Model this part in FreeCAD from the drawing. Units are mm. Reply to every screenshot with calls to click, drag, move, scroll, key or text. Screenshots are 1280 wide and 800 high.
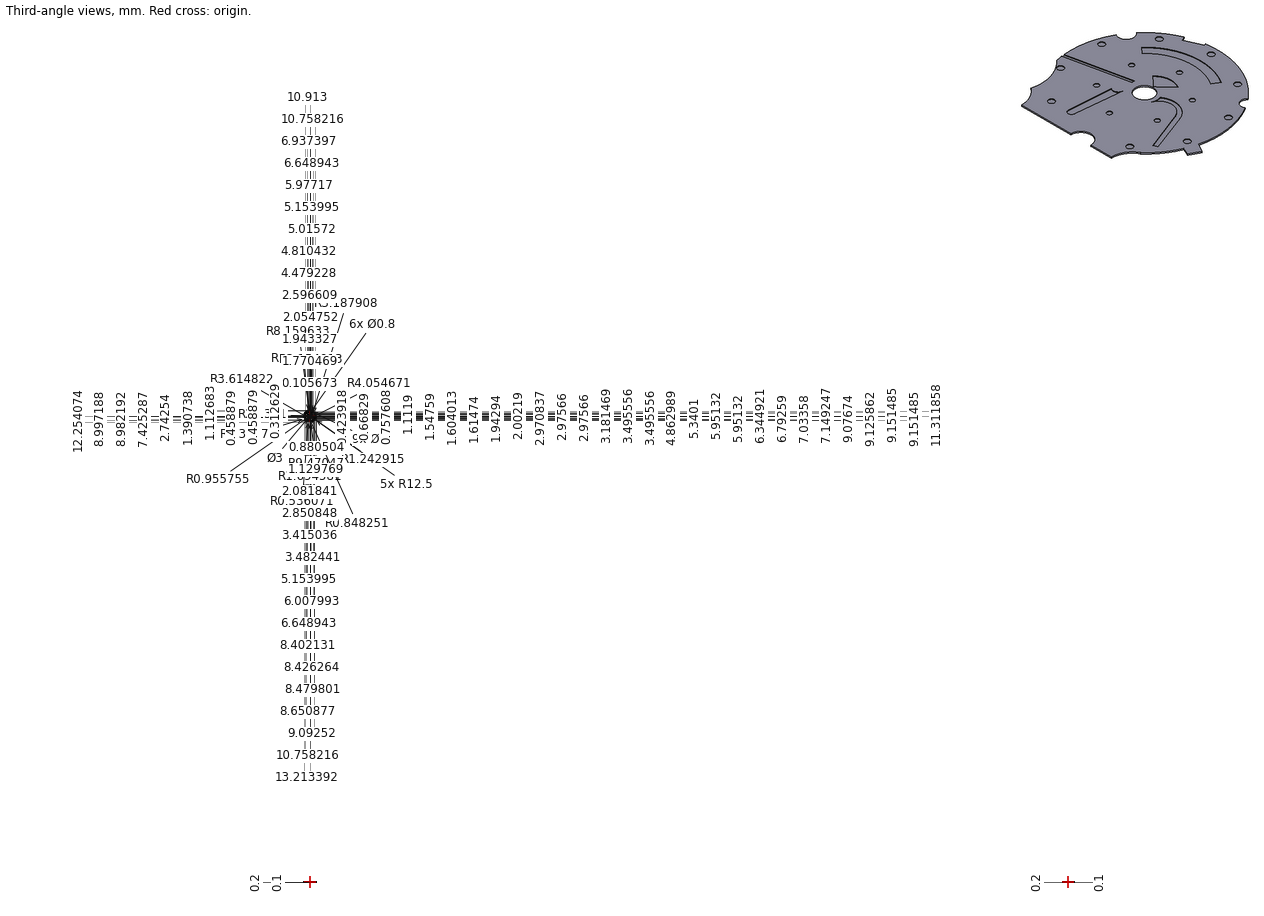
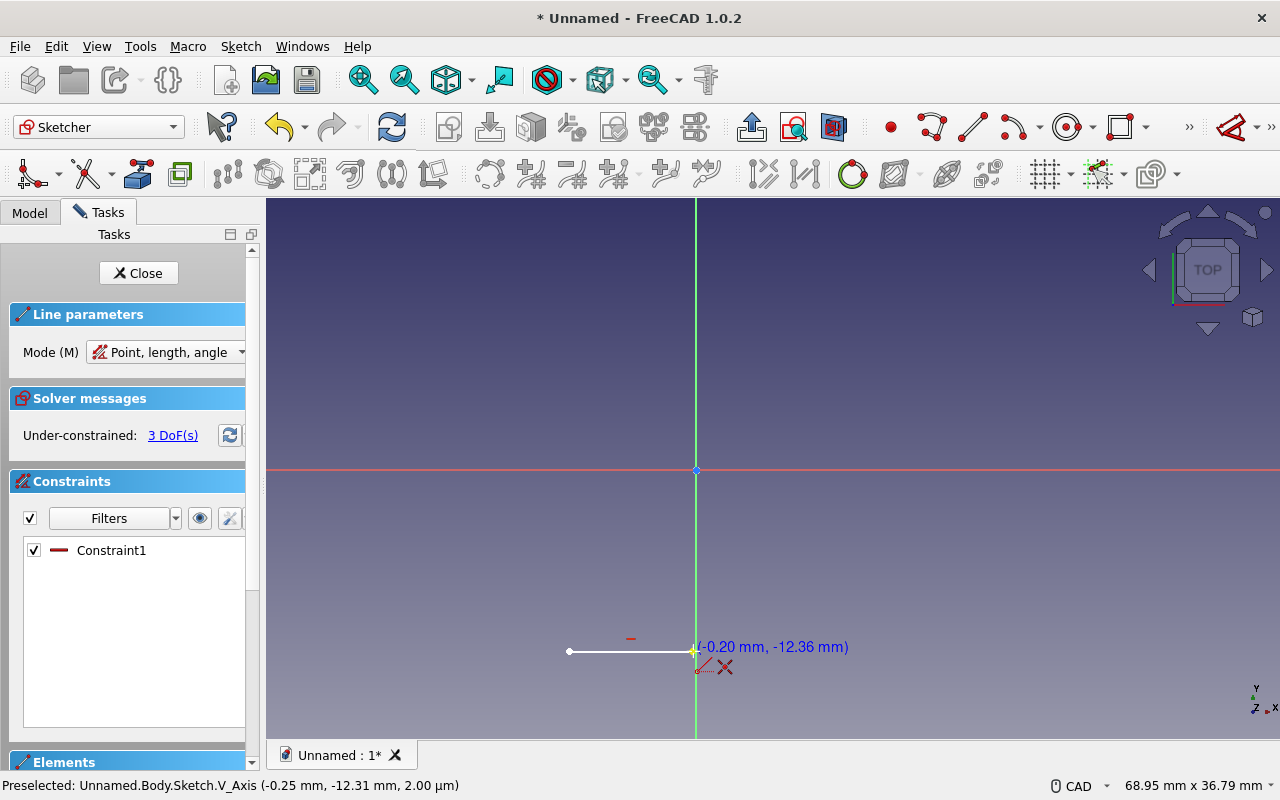
click(743, 650)
click(794, 650)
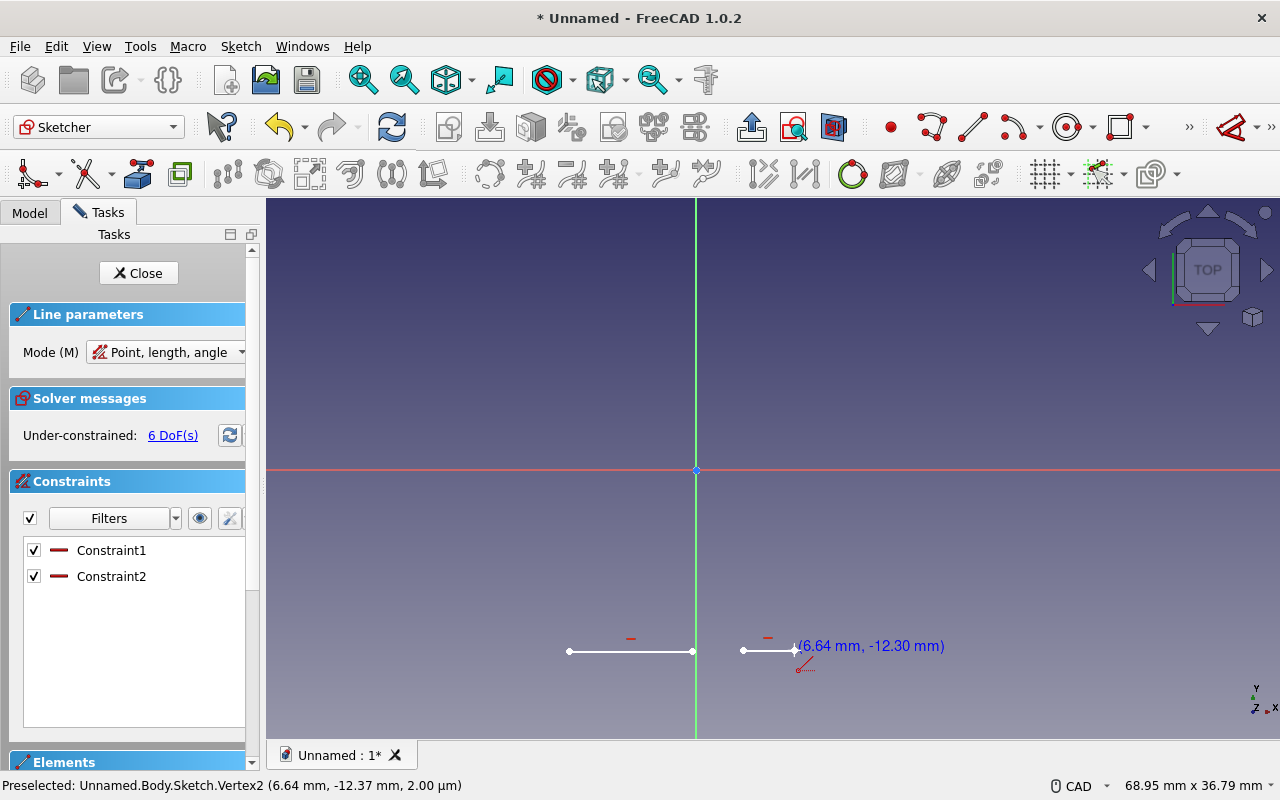
click(820, 604)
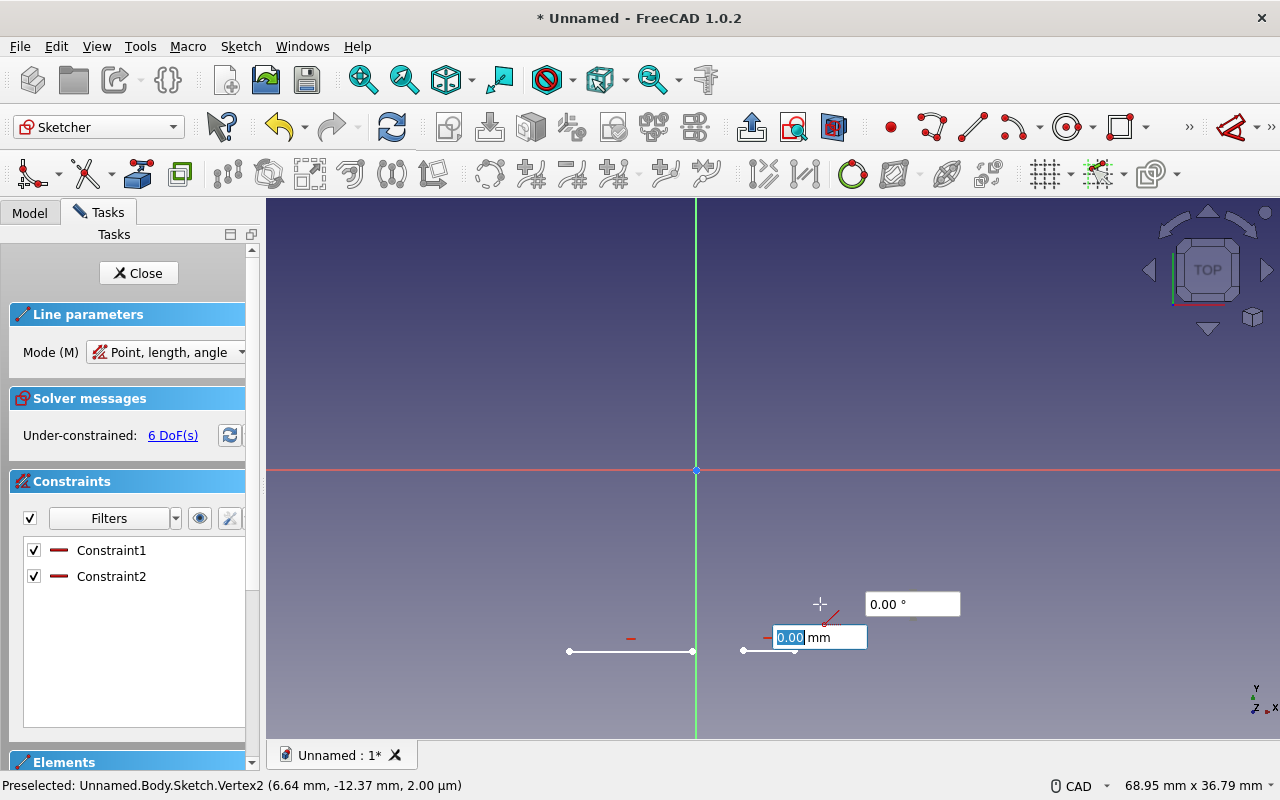
scroll(821, 605, up, 14)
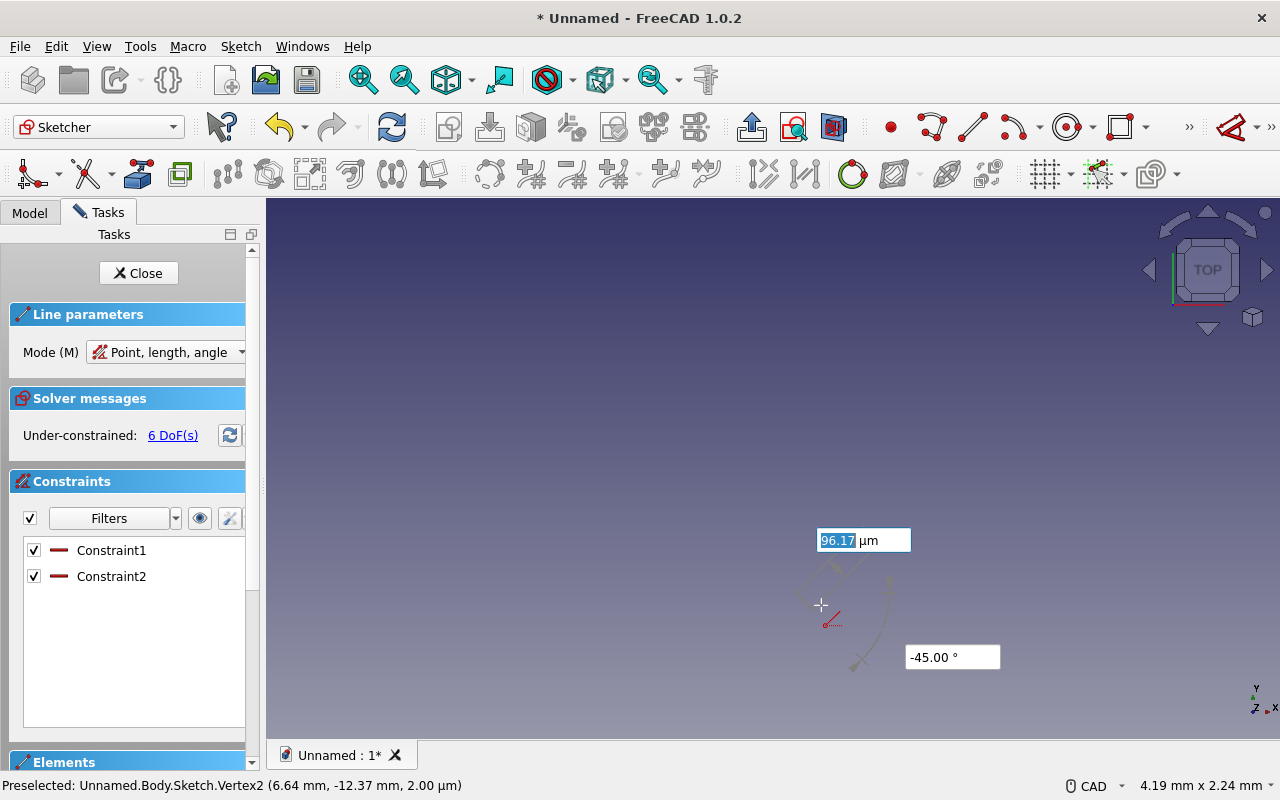
click(813, 596)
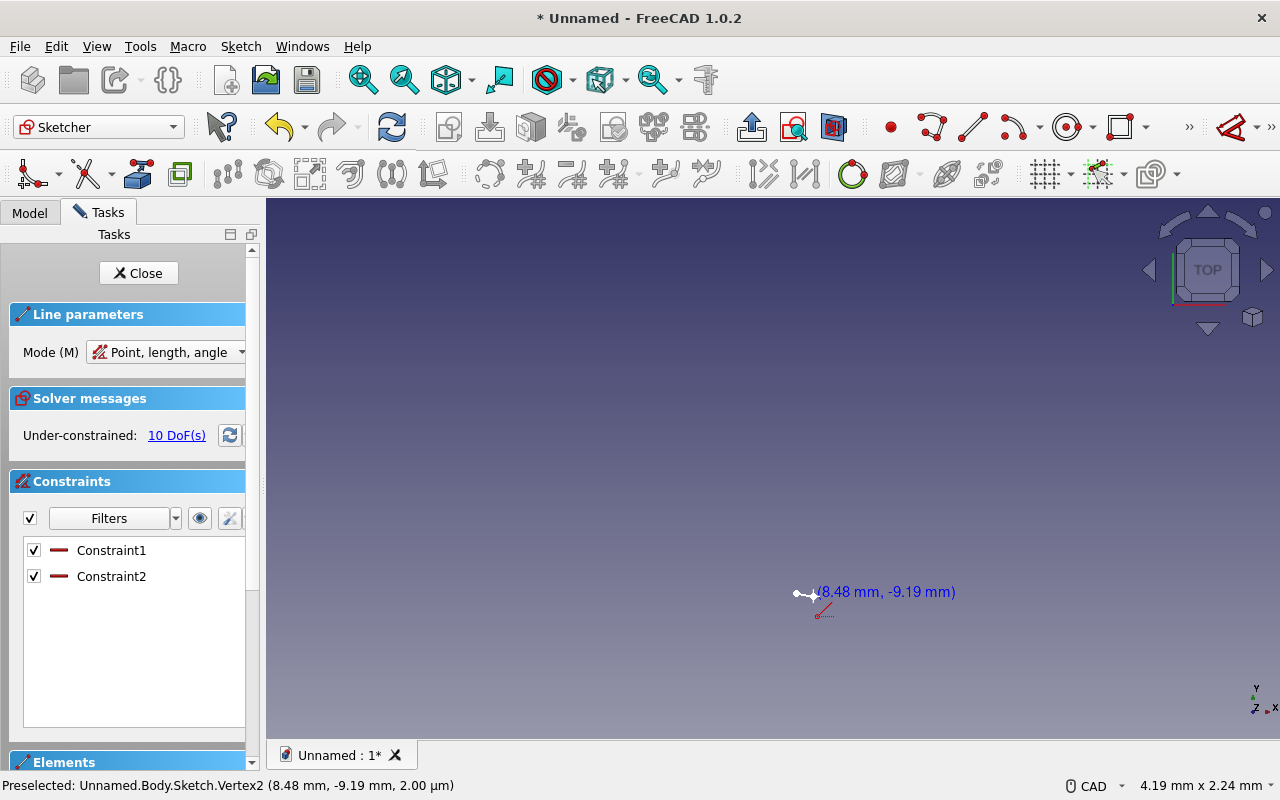
click(932, 128)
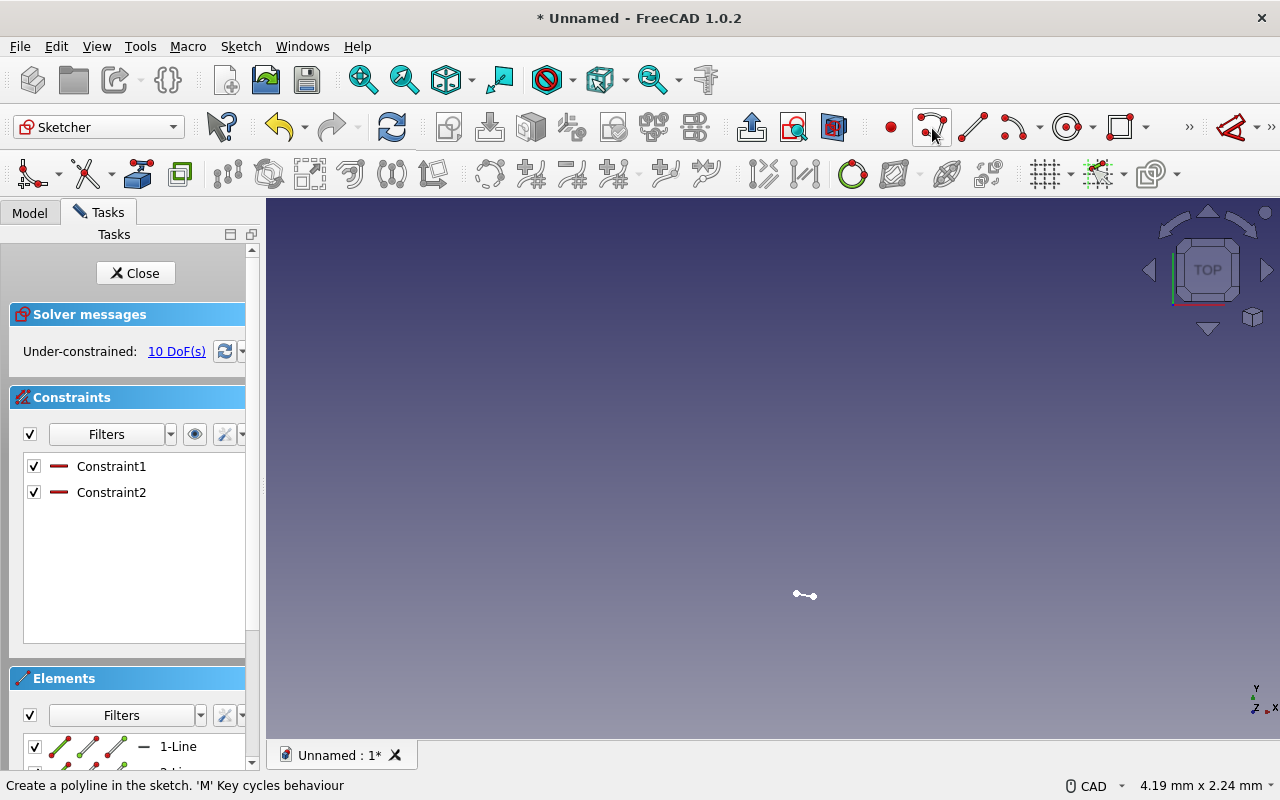
scroll(821, 605, down, 14)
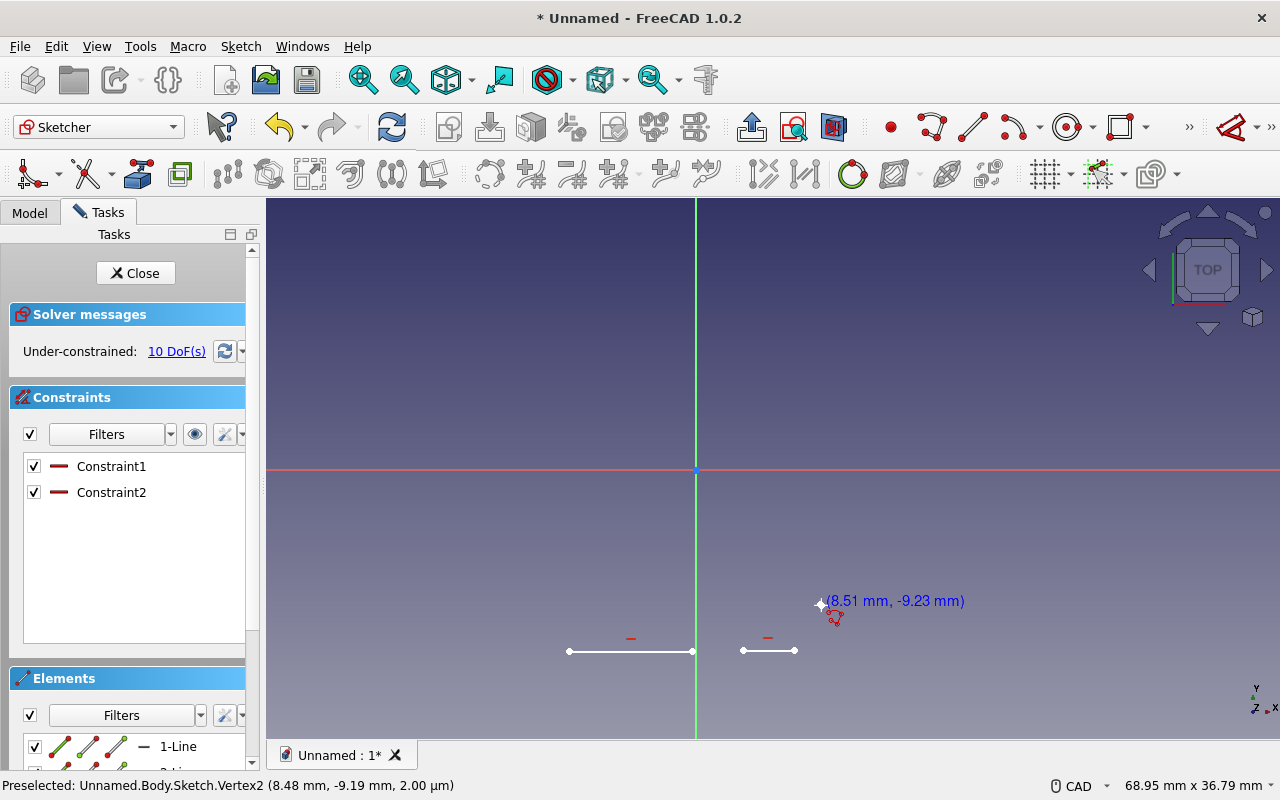
click(866, 542)
click(882, 549)
click(895, 525)
click(875, 514)
right_click(875, 514)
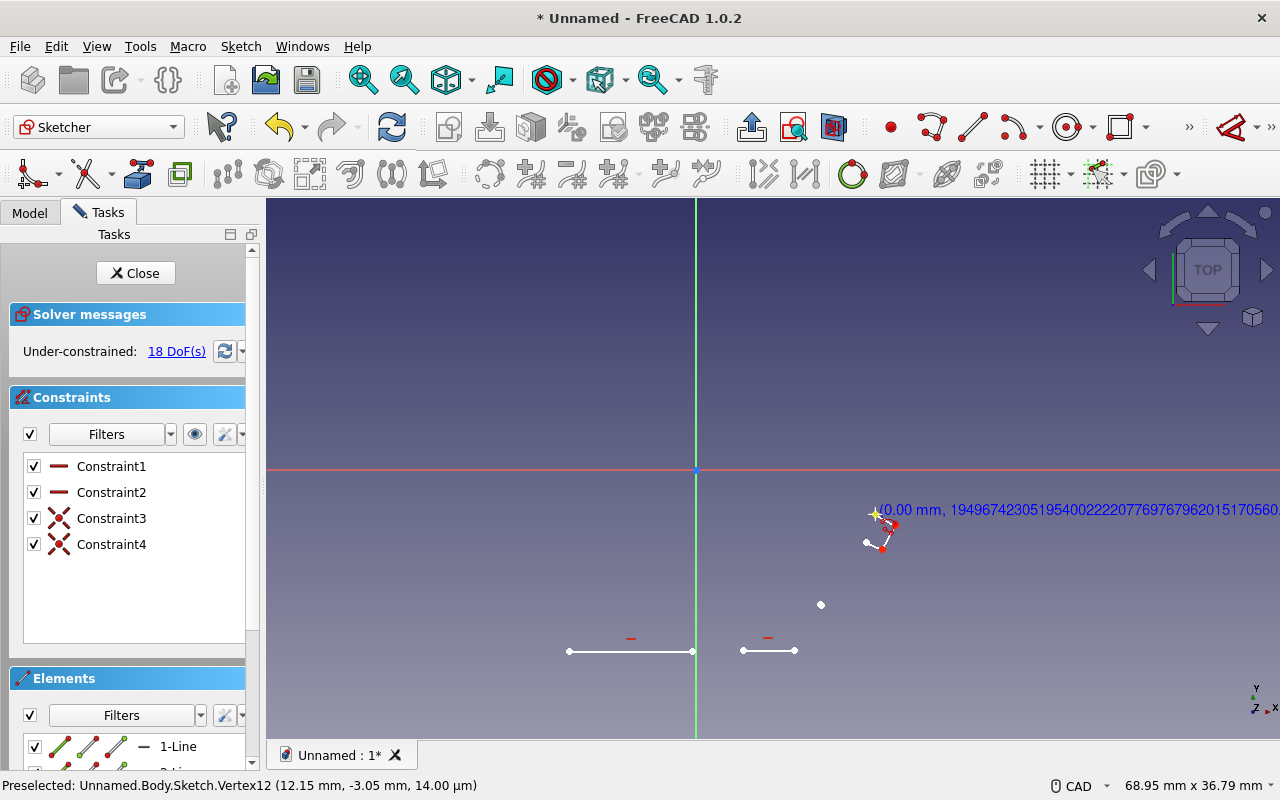
click(668, 289)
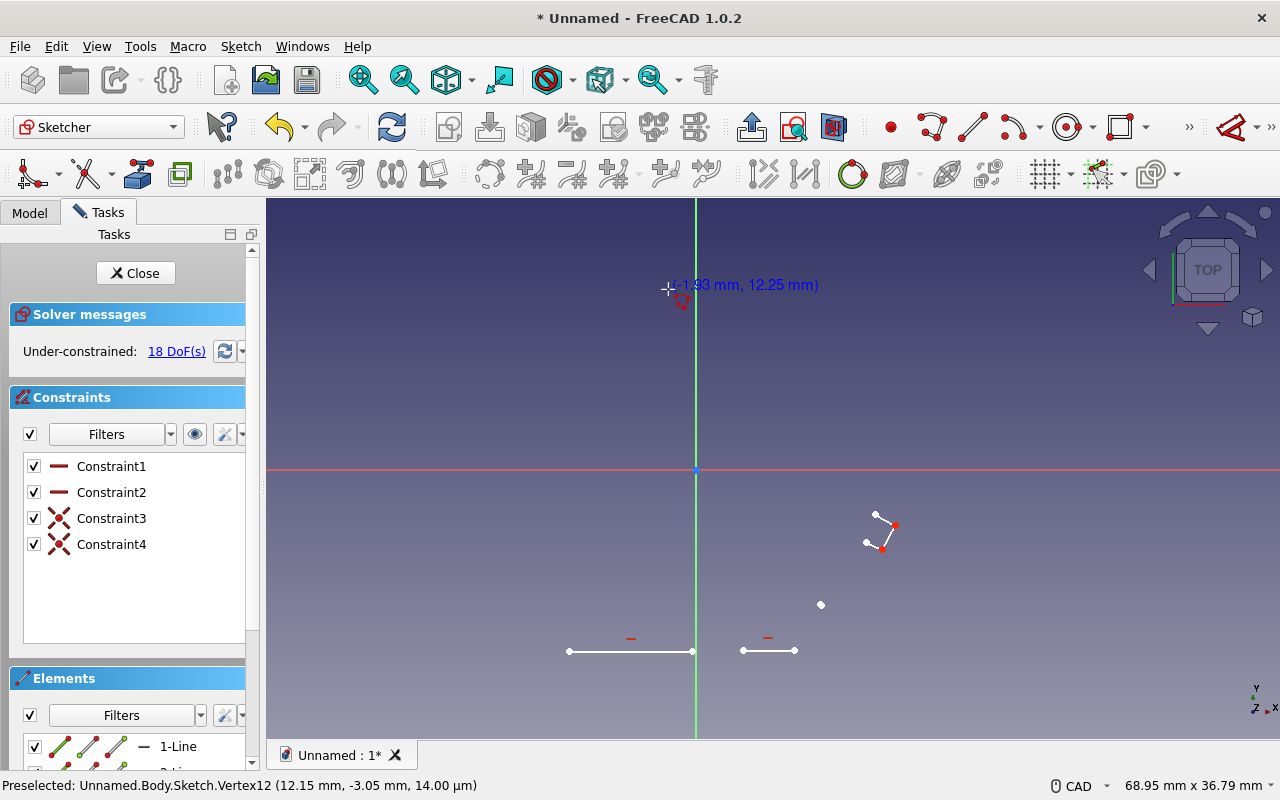
scroll(668, 293, up, 7)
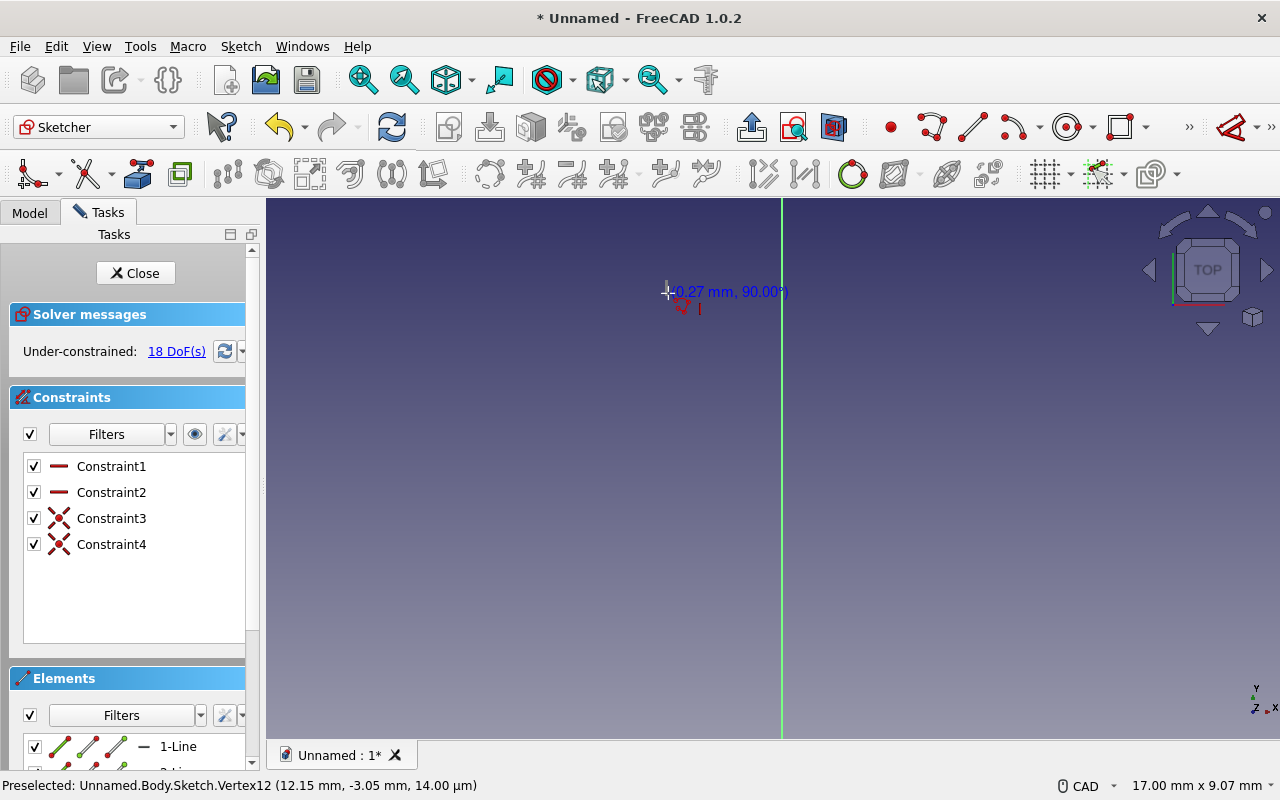
click(667, 293)